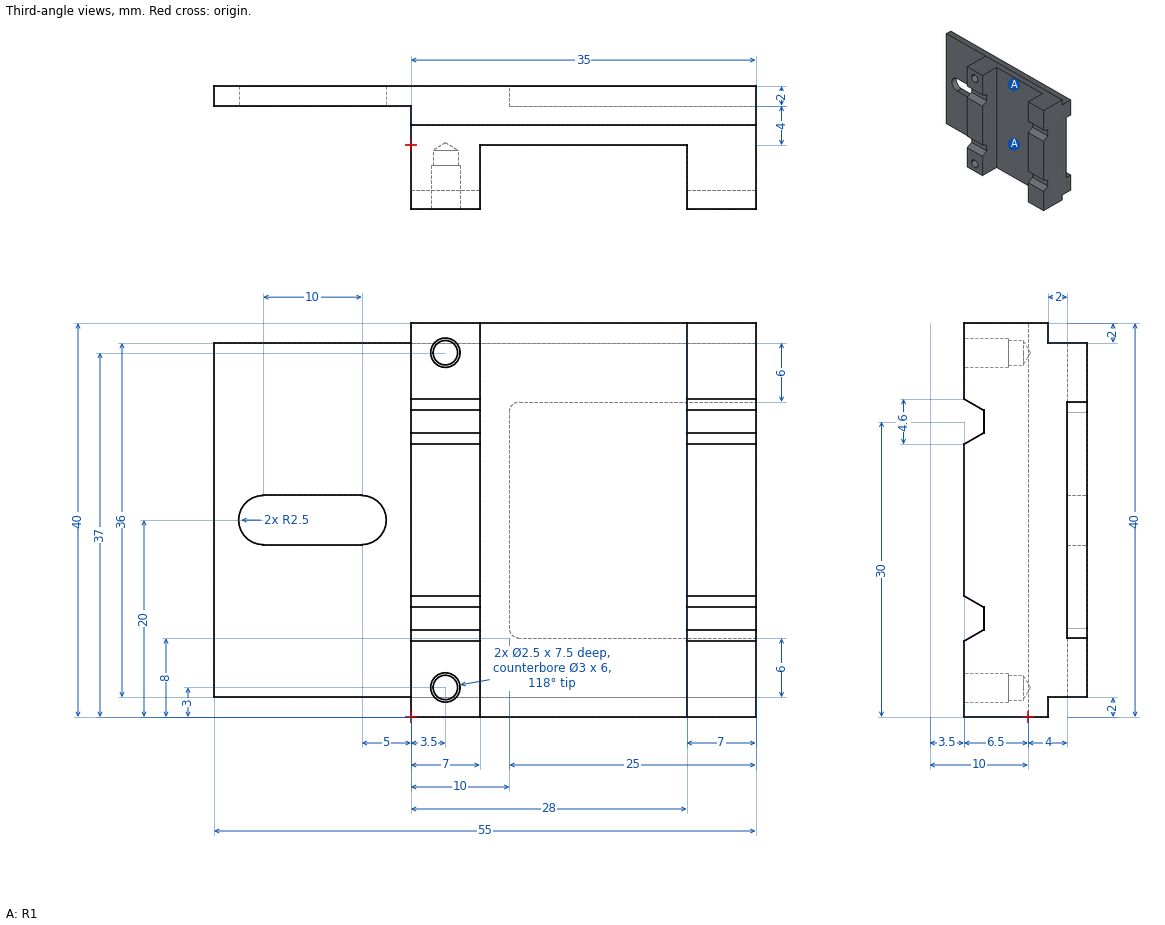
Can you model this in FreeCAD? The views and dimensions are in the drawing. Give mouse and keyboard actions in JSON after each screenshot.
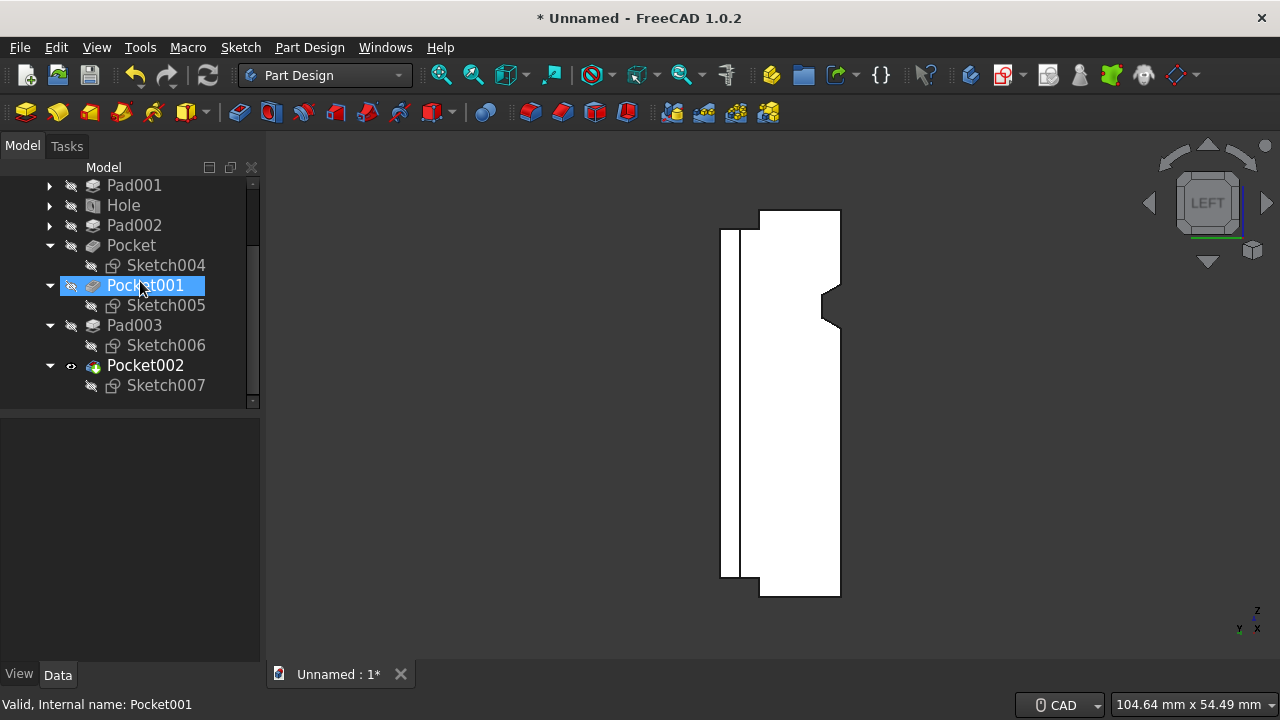
{"action": "scroll", "coordinate": [140, 281], "scroll_direction": "up", "scroll_amount": 15}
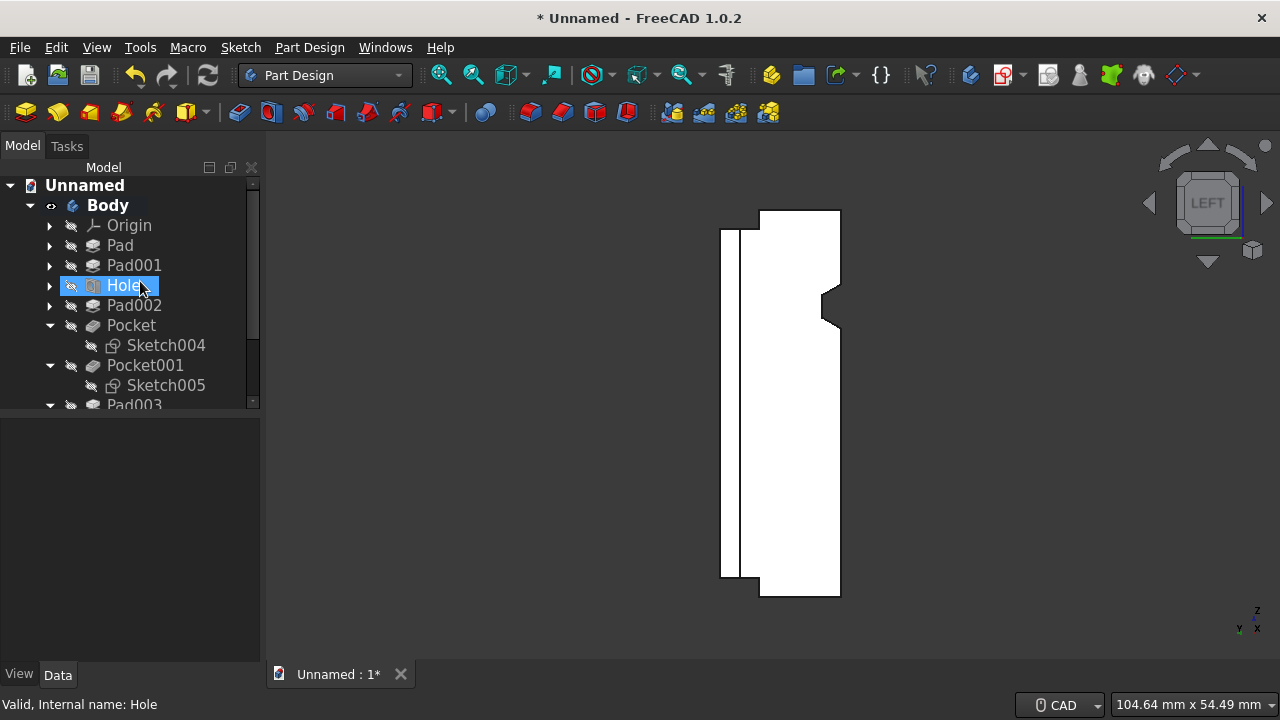
{"action": "left_click", "coordinate": [50, 226]}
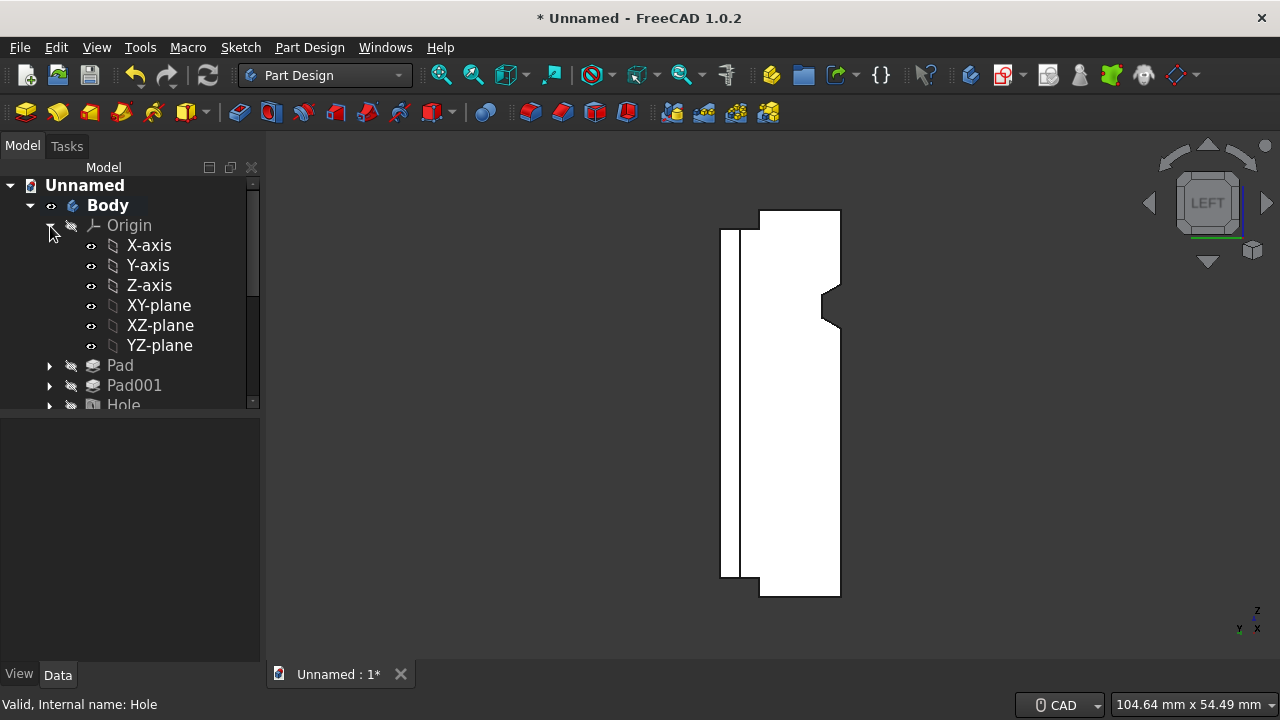
{"action": "left_click", "coordinate": [136, 306]}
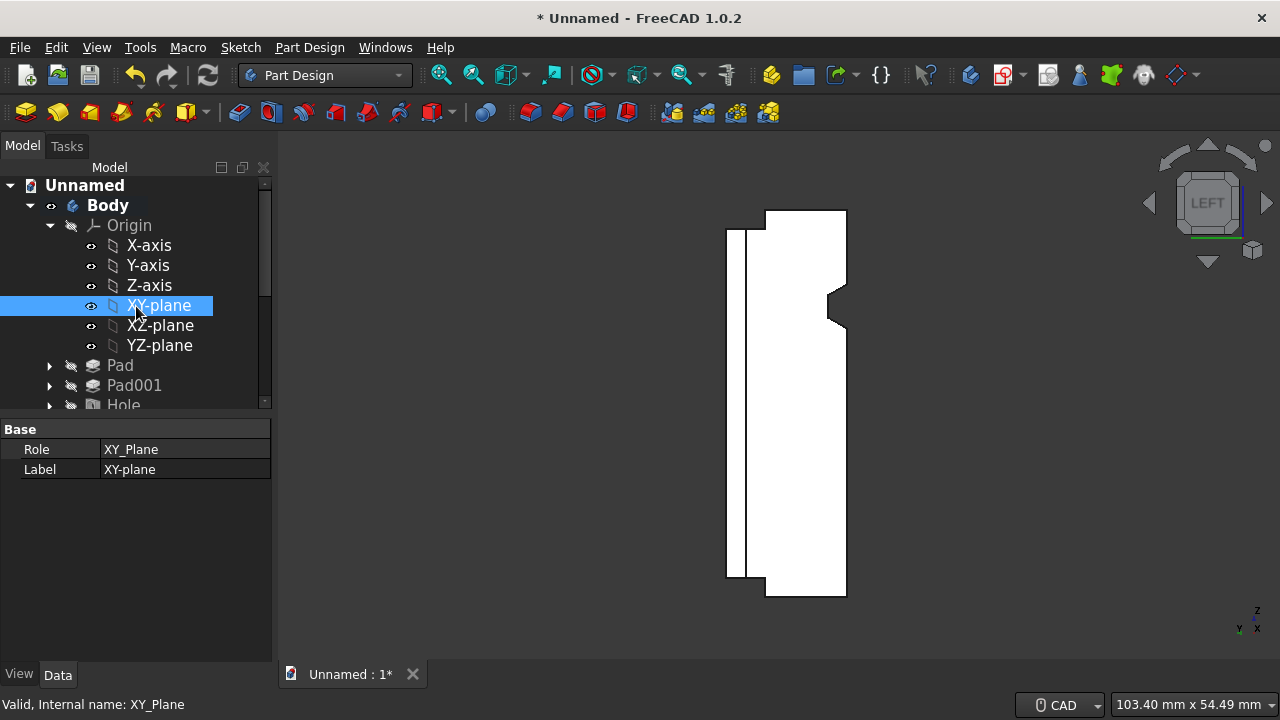
{"action": "left_click", "coordinate": [1176, 76]}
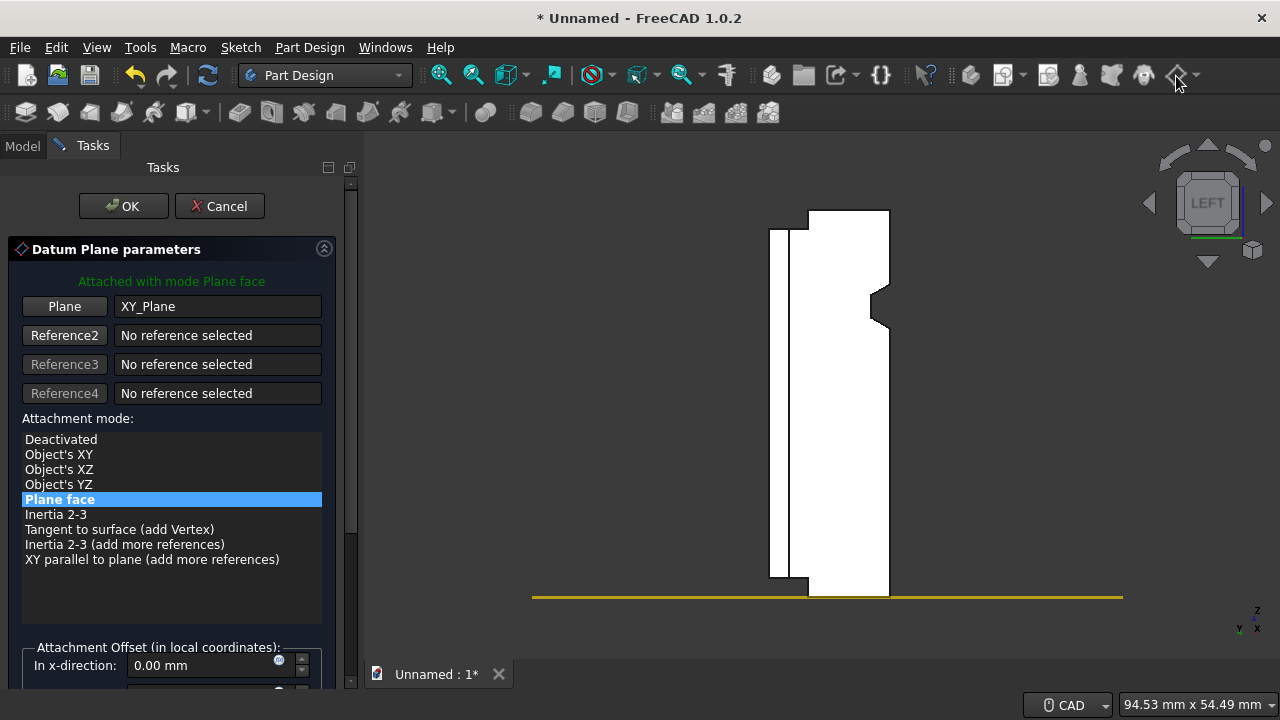
{"action": "scroll", "coordinate": [351, 432], "scroll_direction": "down", "scroll_amount": 2}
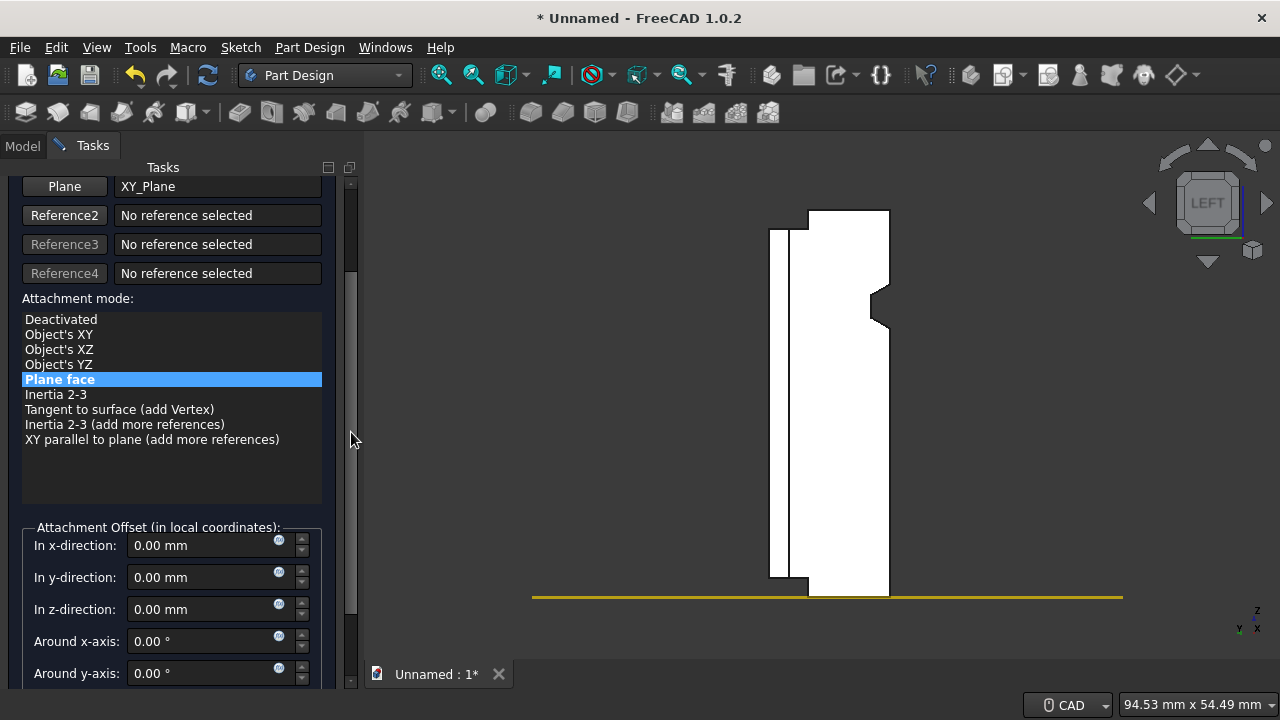
{"action": "triple_click", "coordinate": [210, 609]}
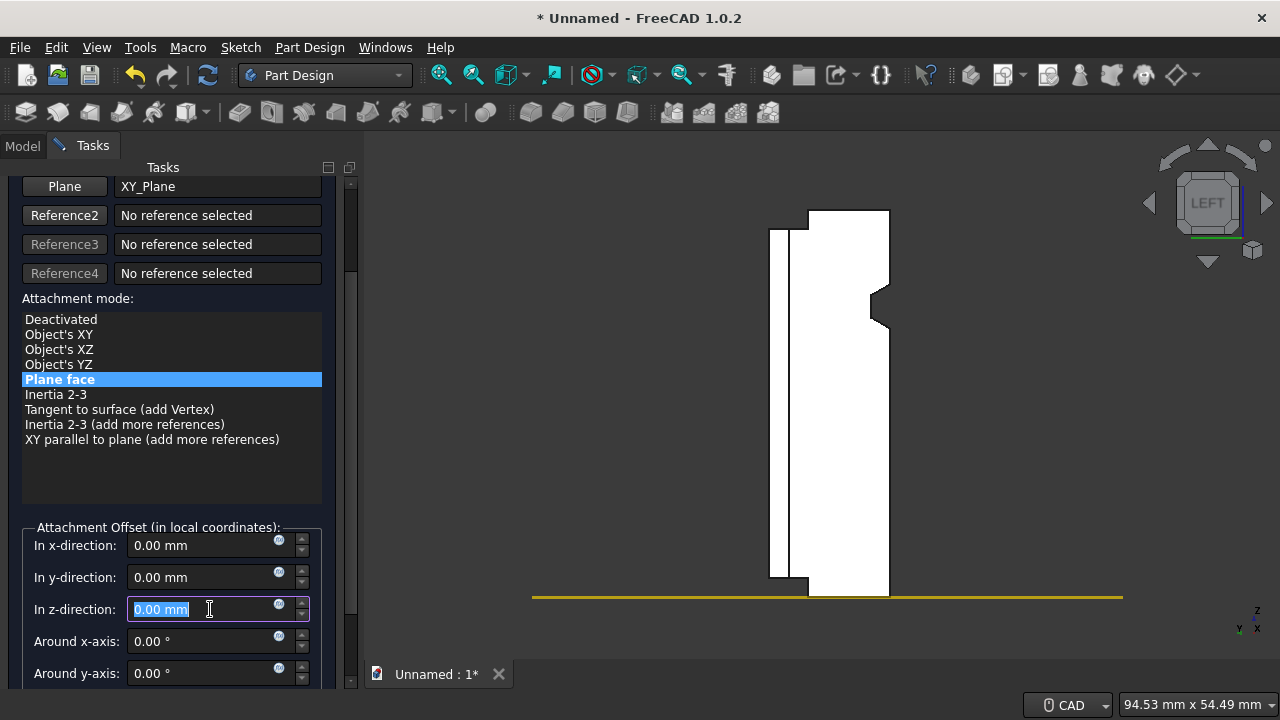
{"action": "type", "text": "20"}
{"action": "key", "text": "Tab"}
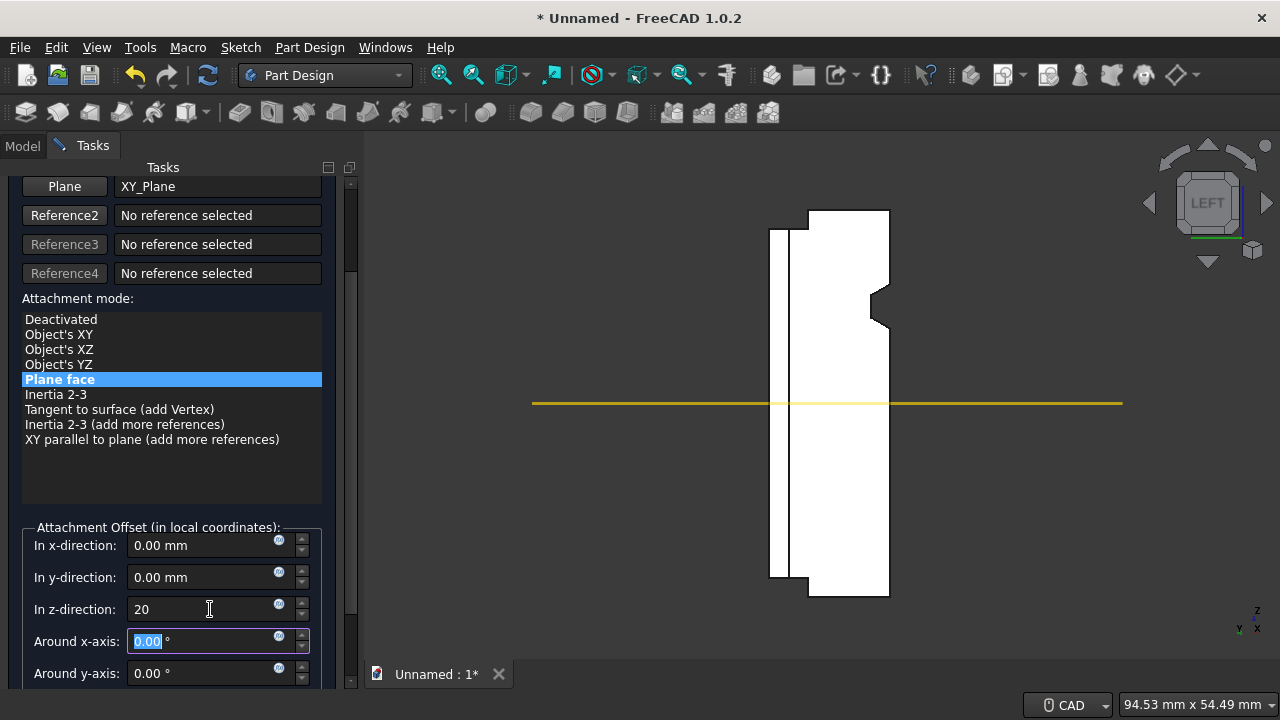
{"action": "scroll", "coordinate": [351, 432], "scroll_direction": "up", "scroll_amount": 3}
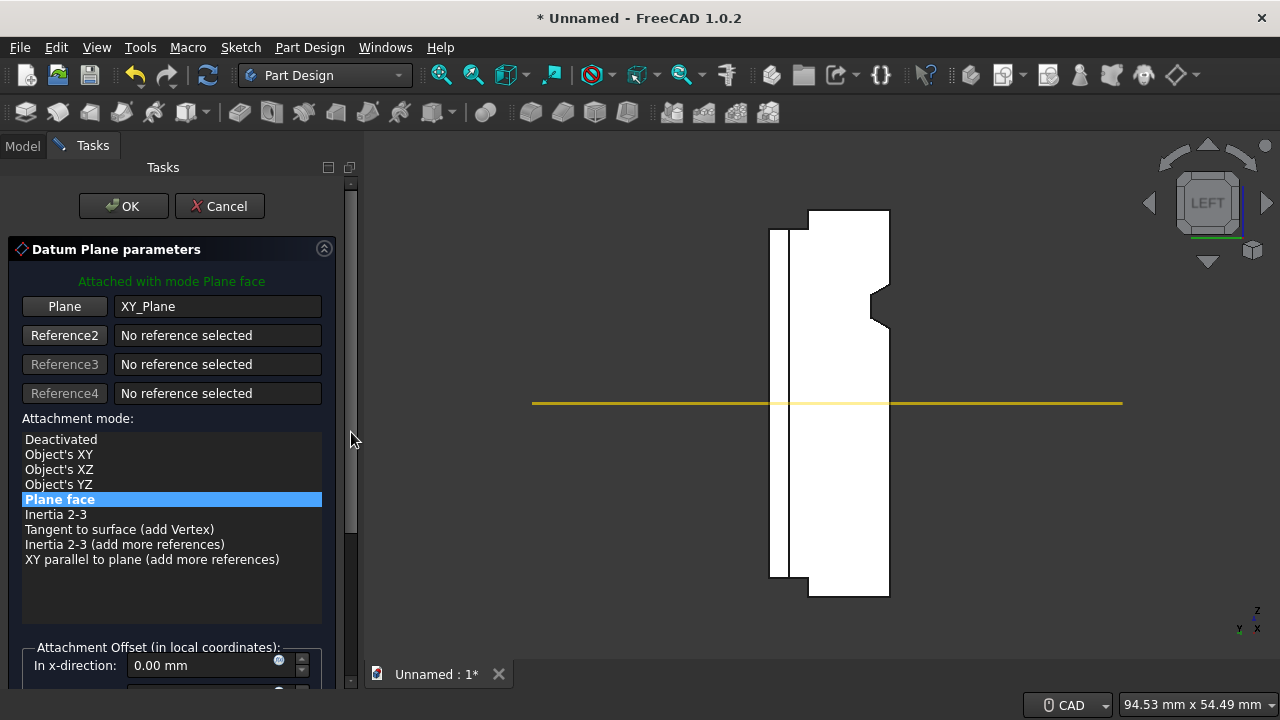
{"action": "left_click", "coordinate": [124, 206]}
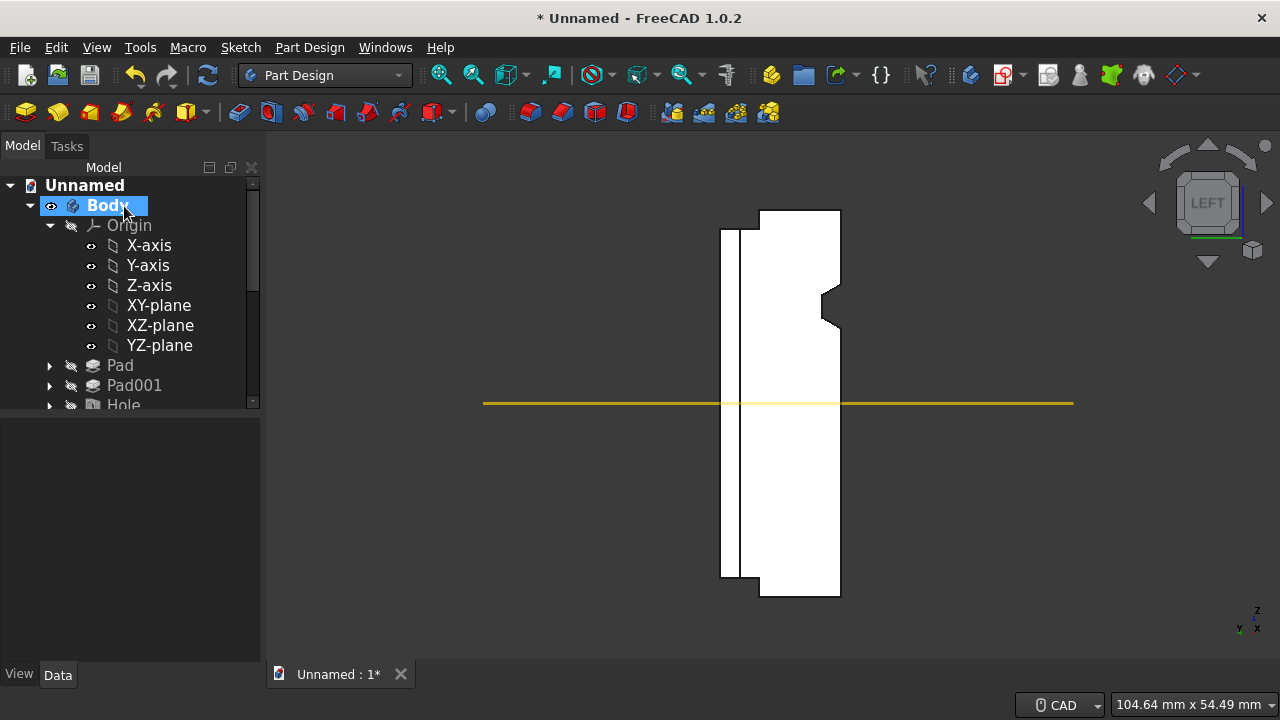
{"action": "scroll", "coordinate": [100, 301], "scroll_direction": "down", "scroll_amount": 3}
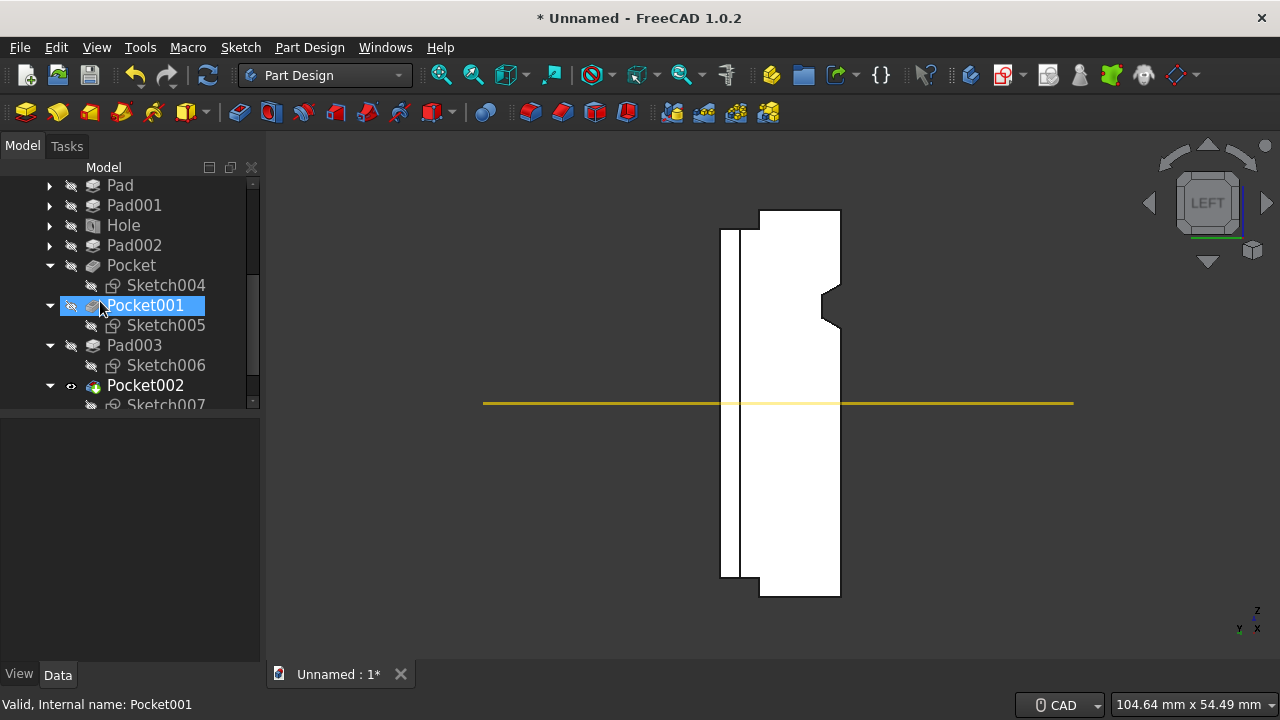
{"action": "left_click", "coordinate": [116, 386]}